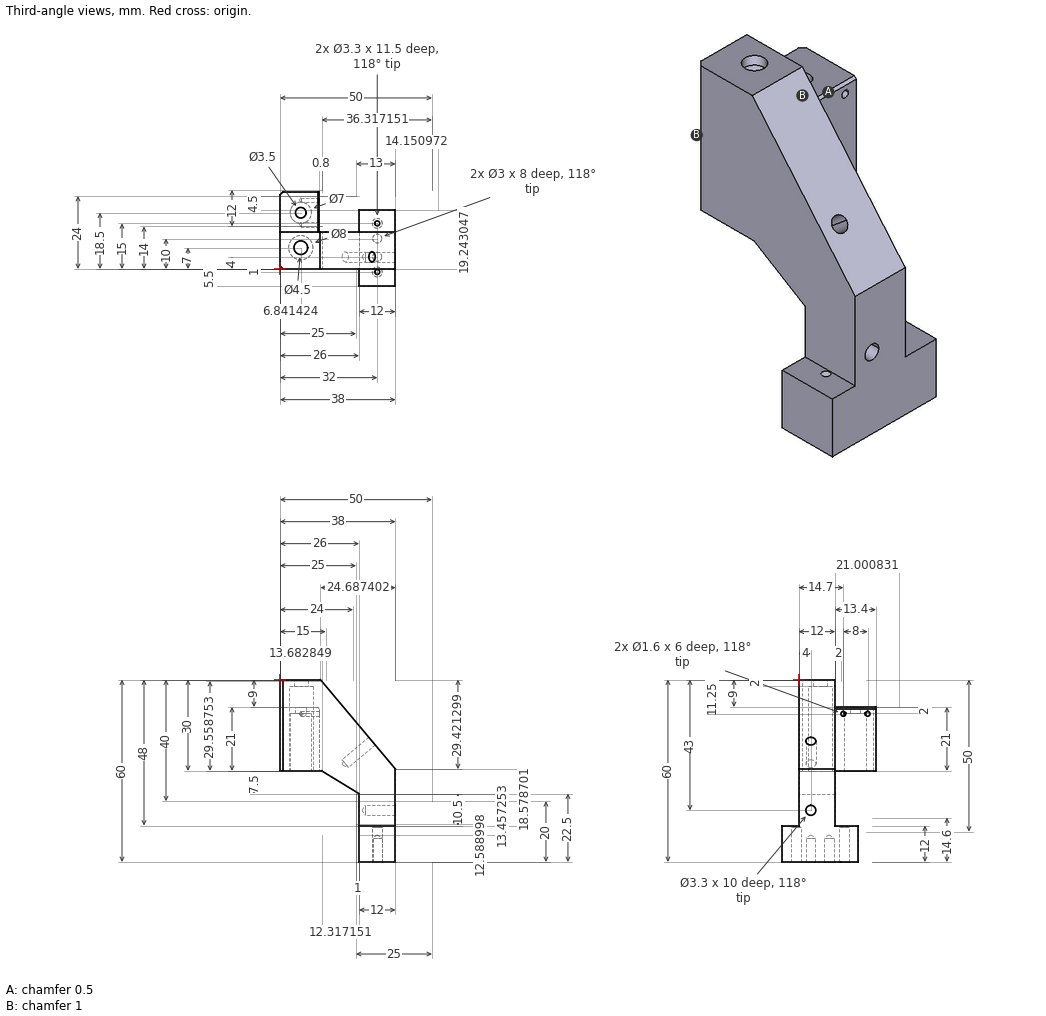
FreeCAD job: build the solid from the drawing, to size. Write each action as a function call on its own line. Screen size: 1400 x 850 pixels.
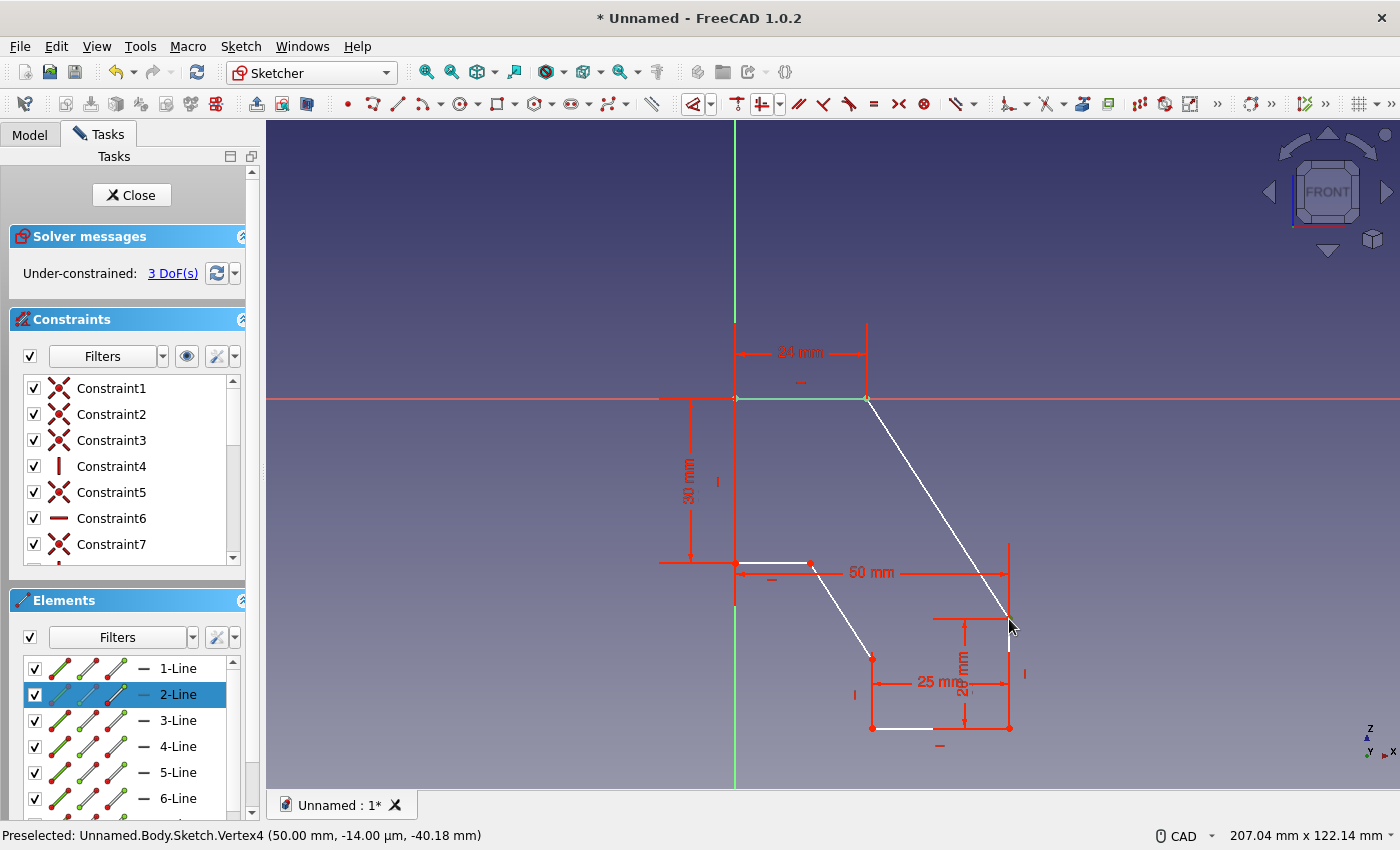
key(i)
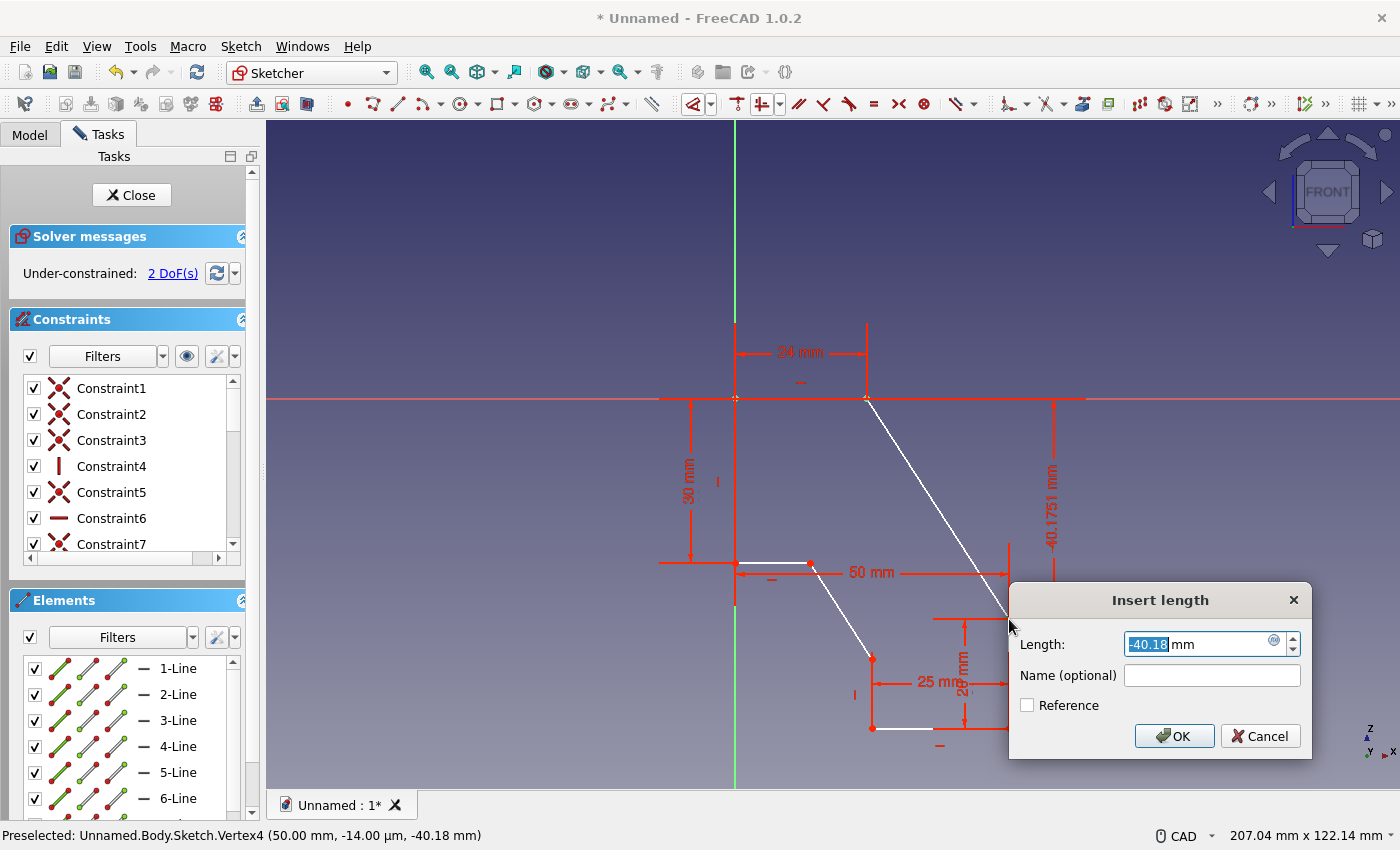
text(-40)
key(Return)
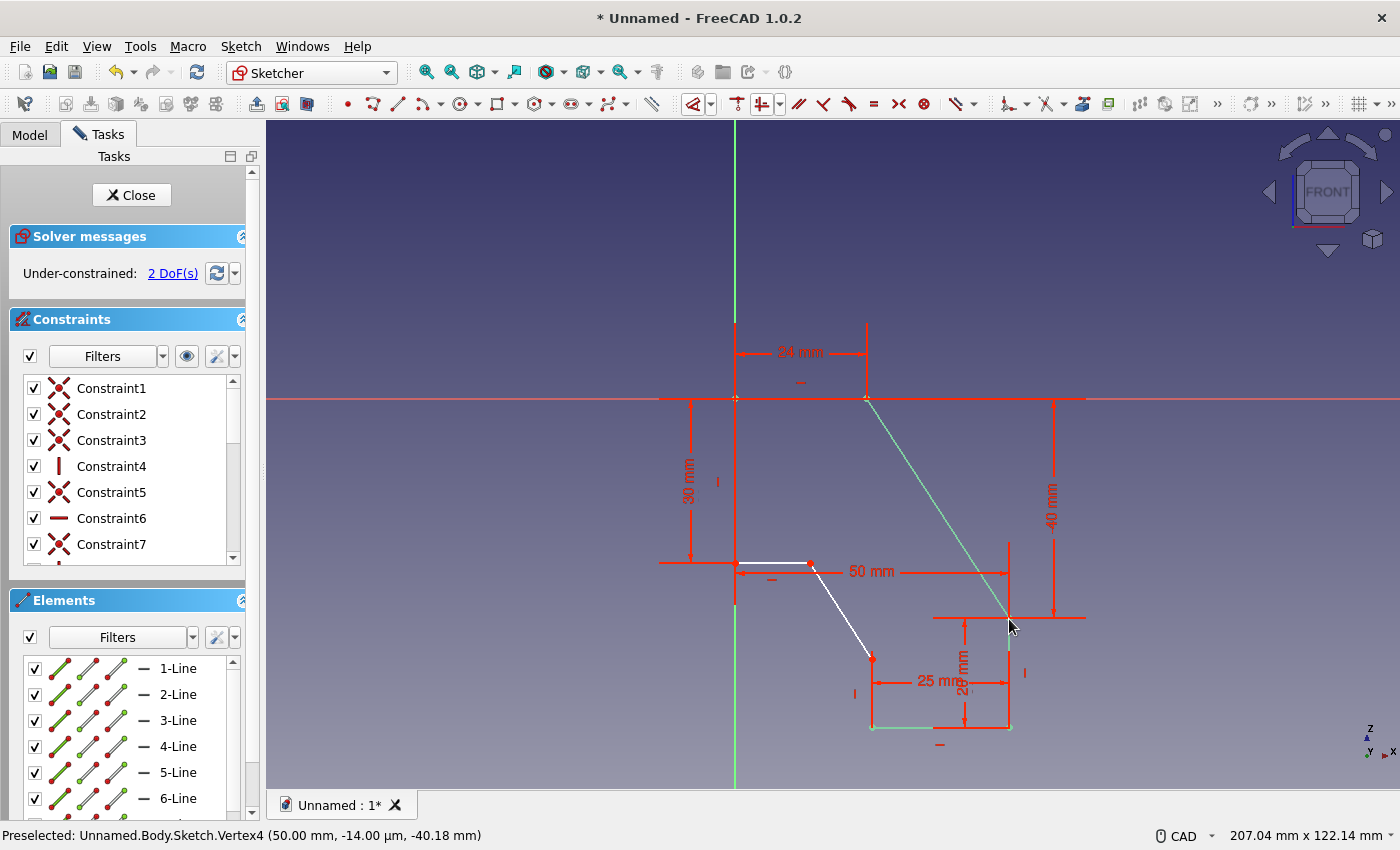
click(872, 707)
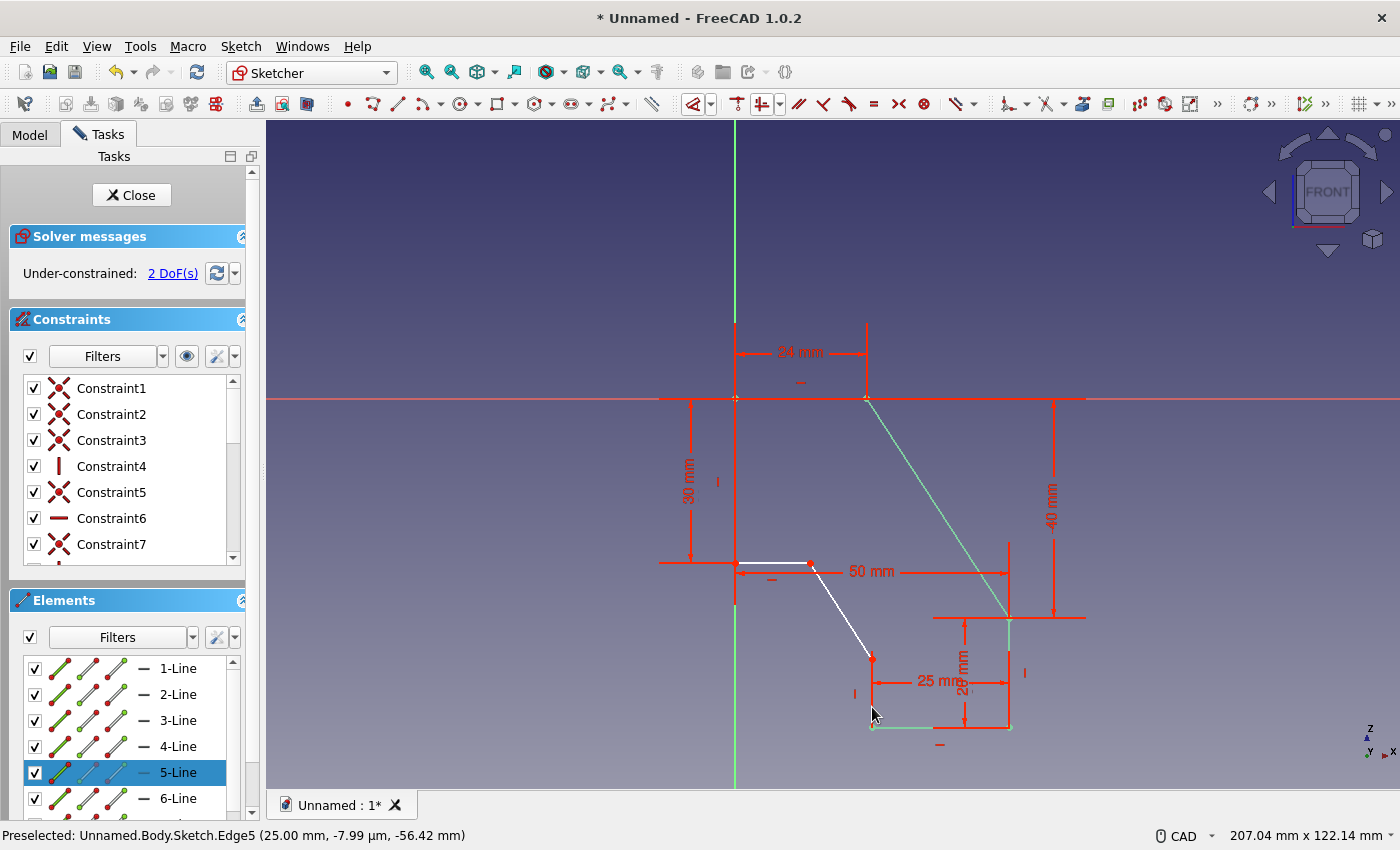
click(710, 104)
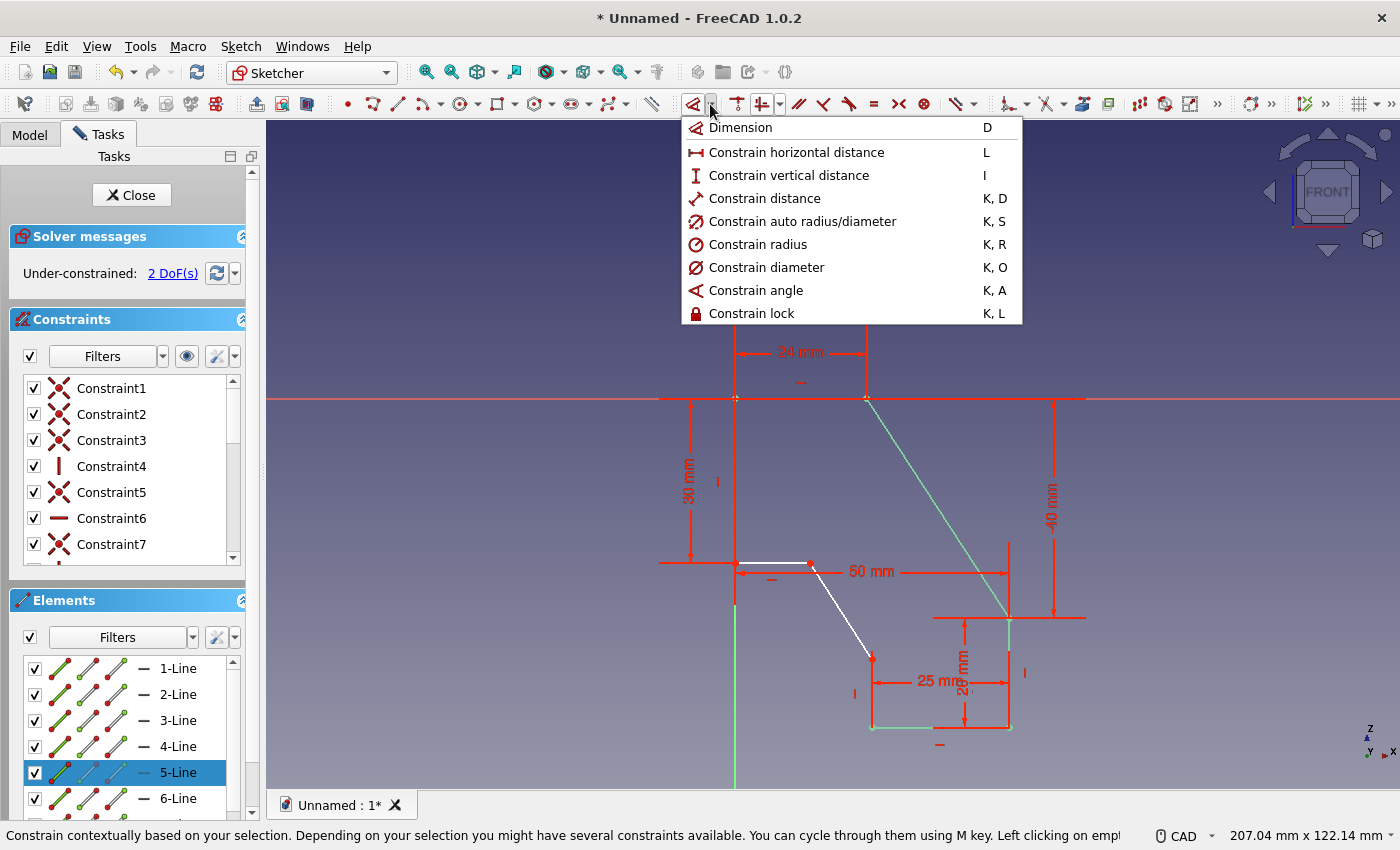
click(852, 176)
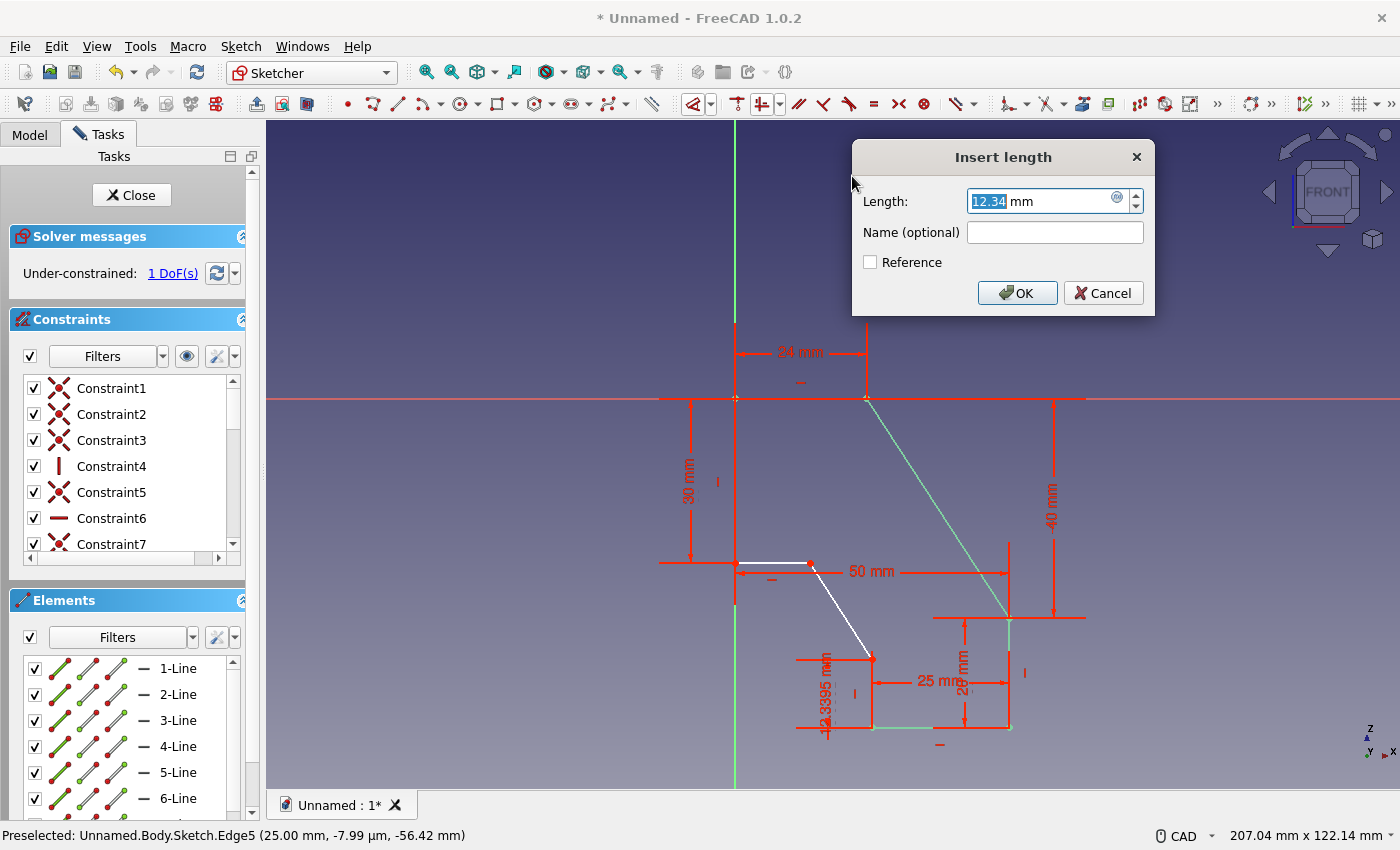
text(12.588998)
key(Return)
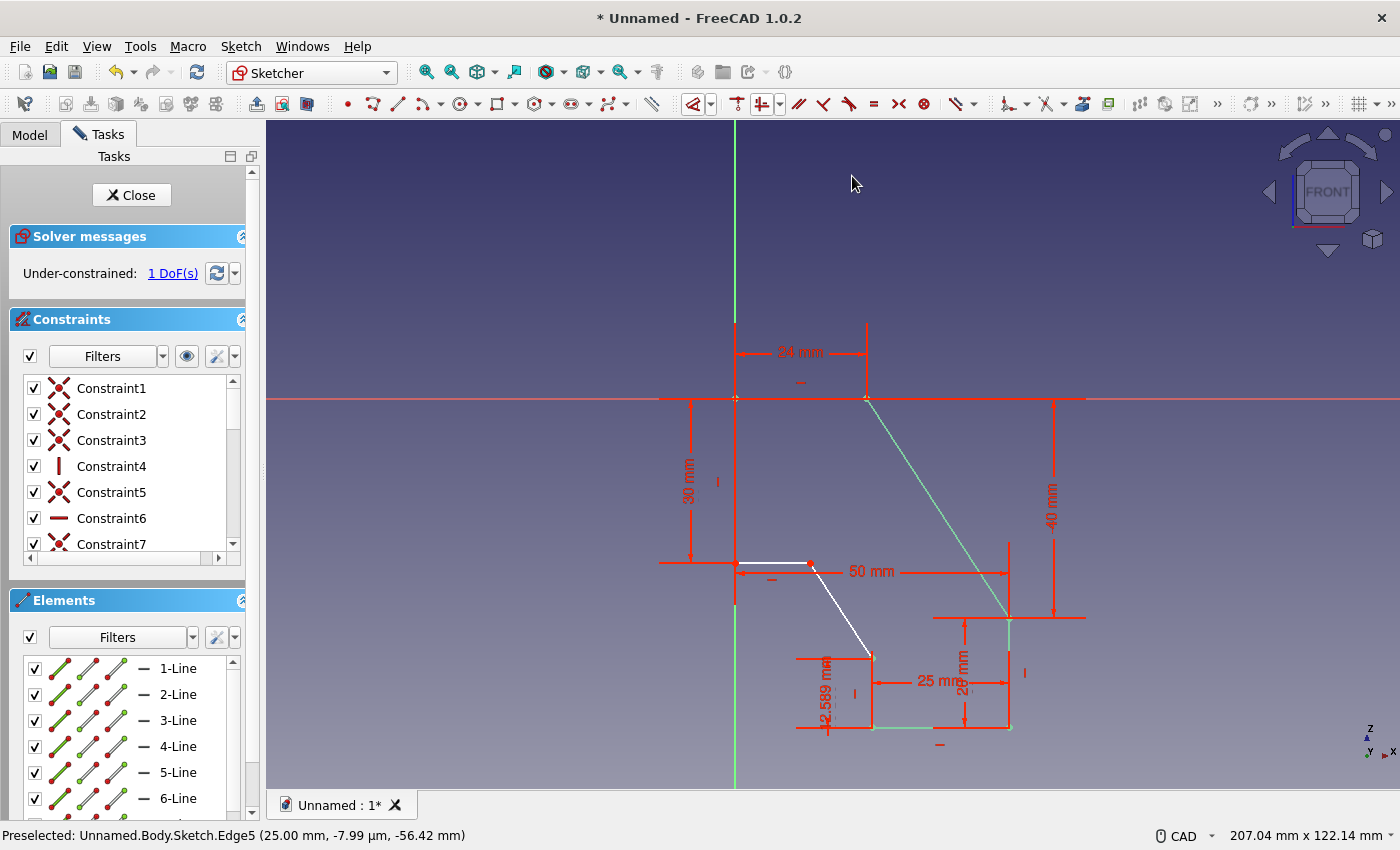
click(788, 563)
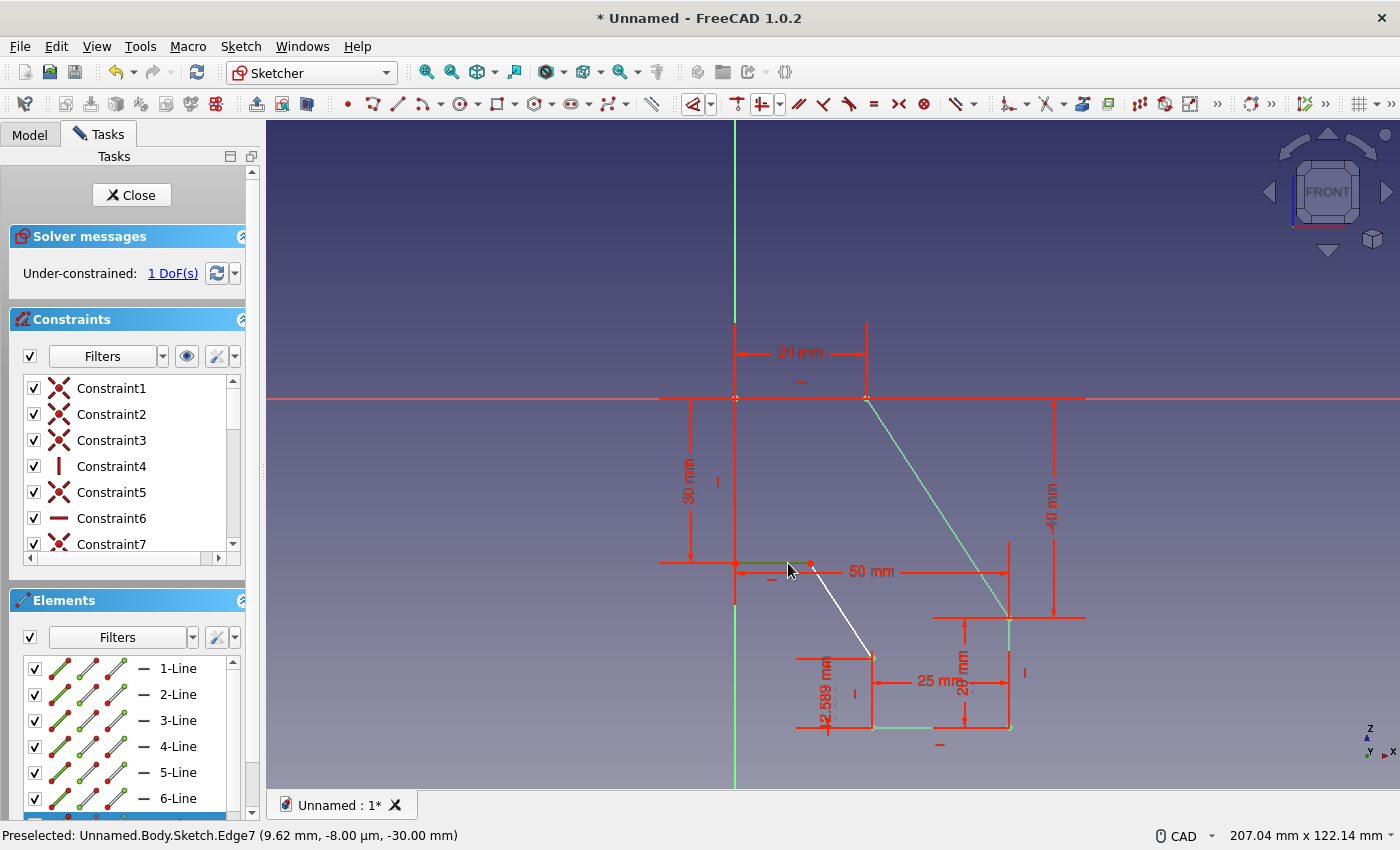
key(l)